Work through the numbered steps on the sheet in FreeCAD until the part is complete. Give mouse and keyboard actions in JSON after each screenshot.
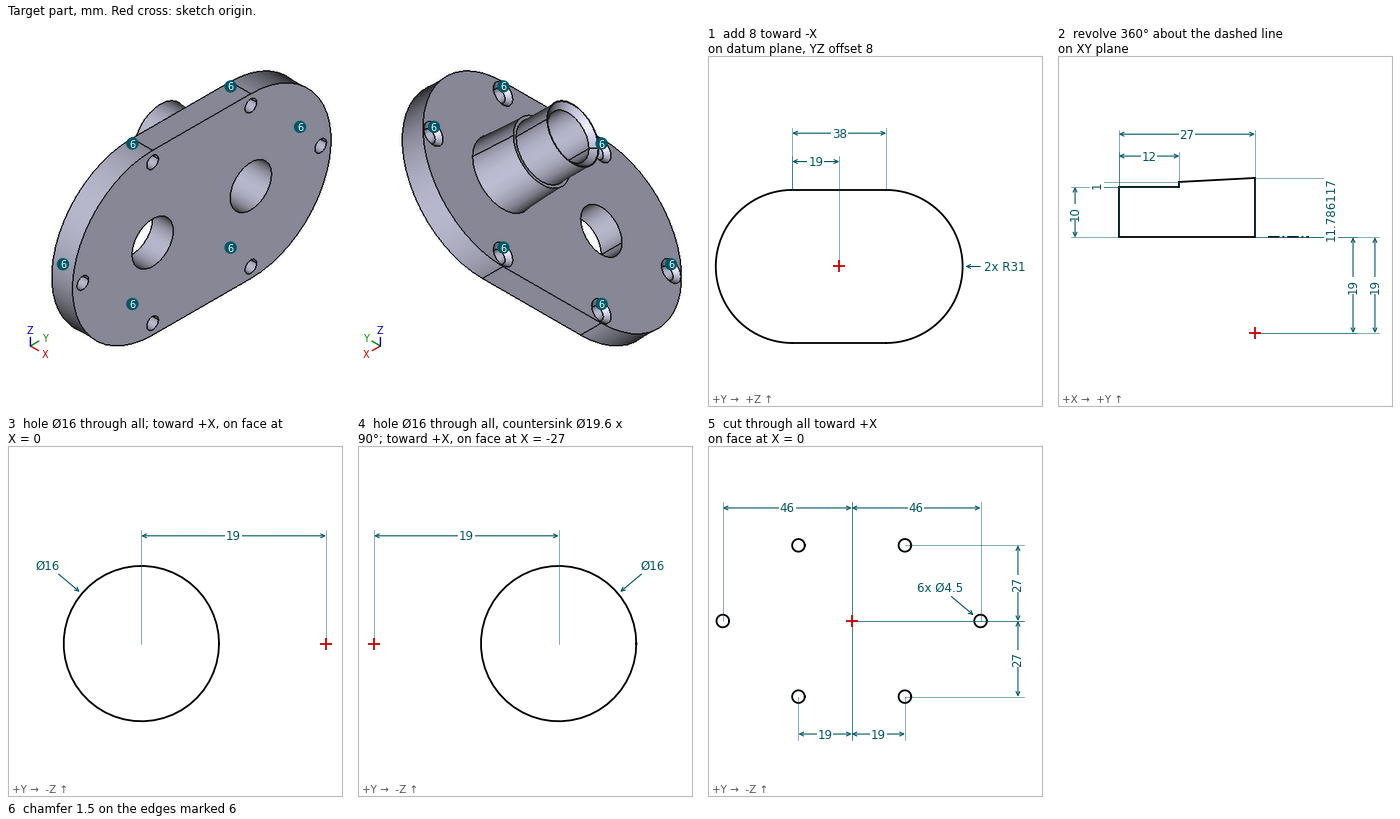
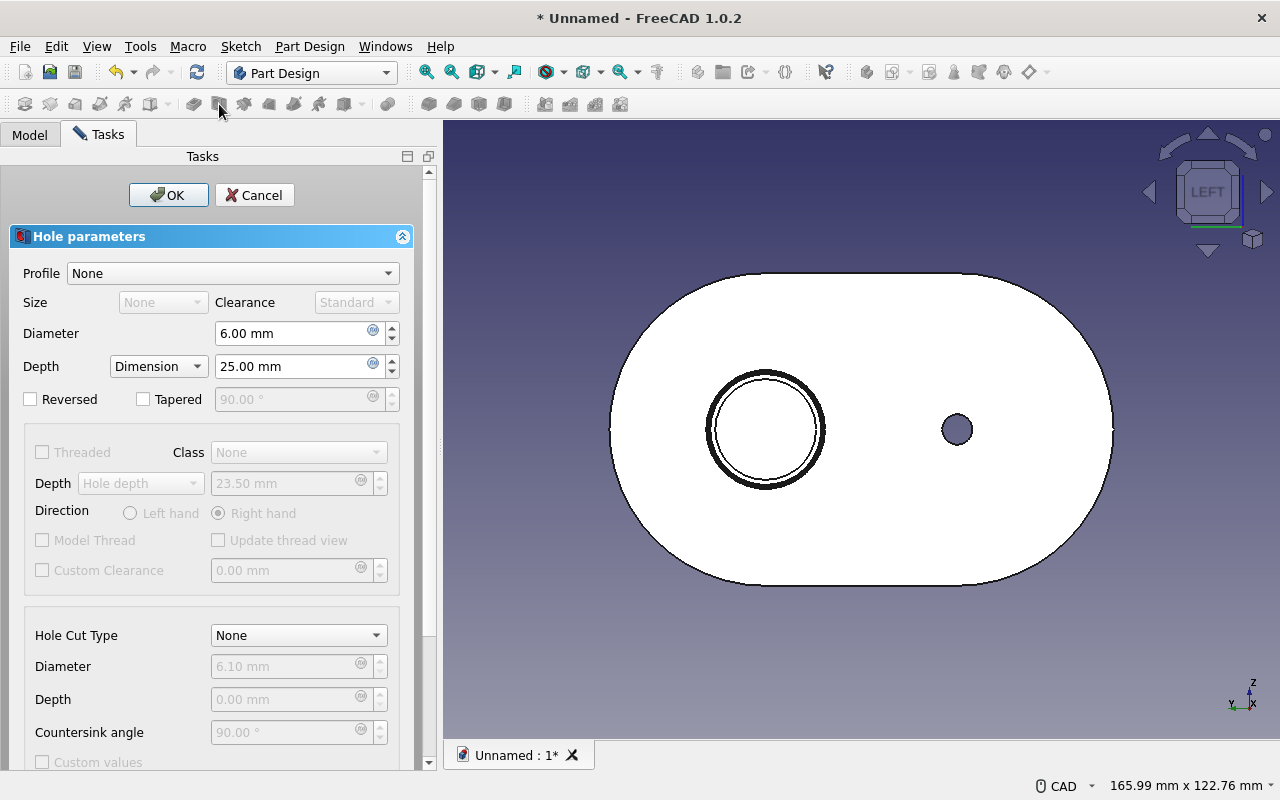
{"action": "triple_click", "coordinate": [300, 334]}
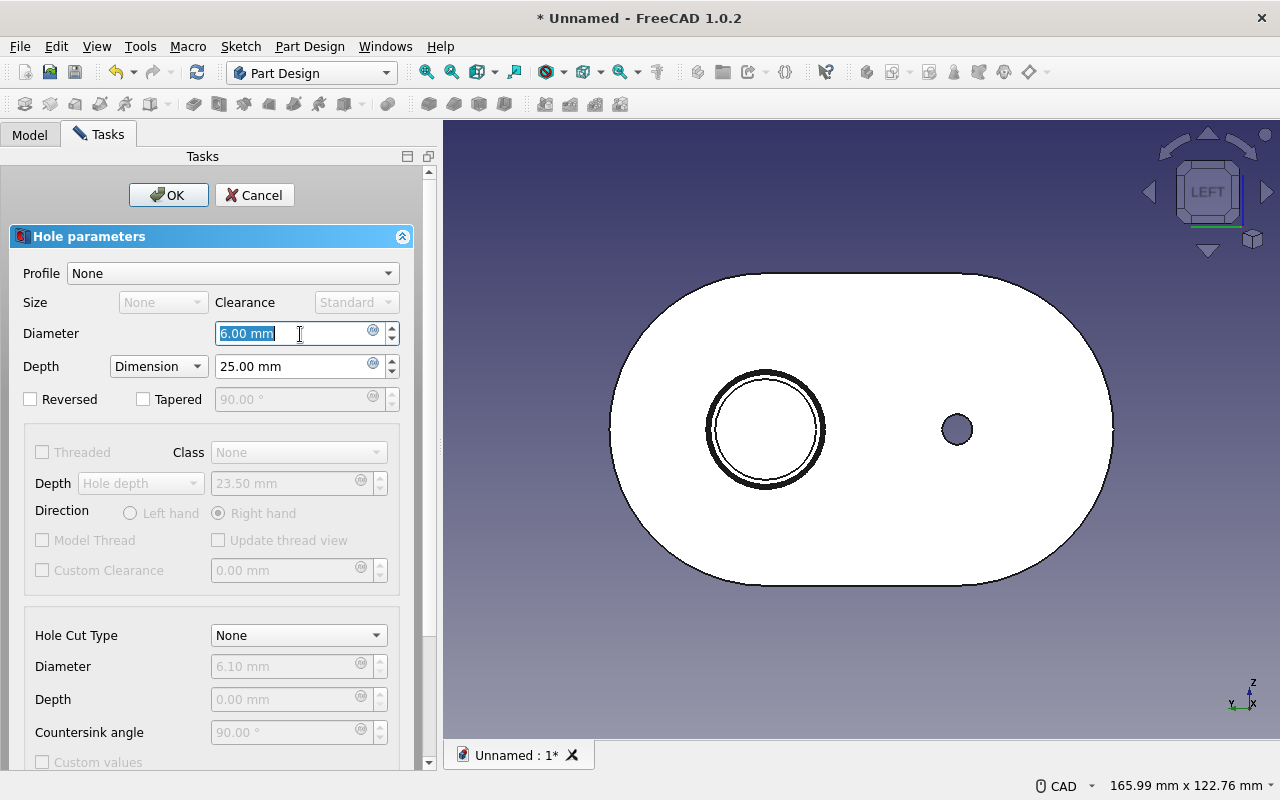
{"action": "type", "text": "16"}
{"action": "key", "text": "Tab"}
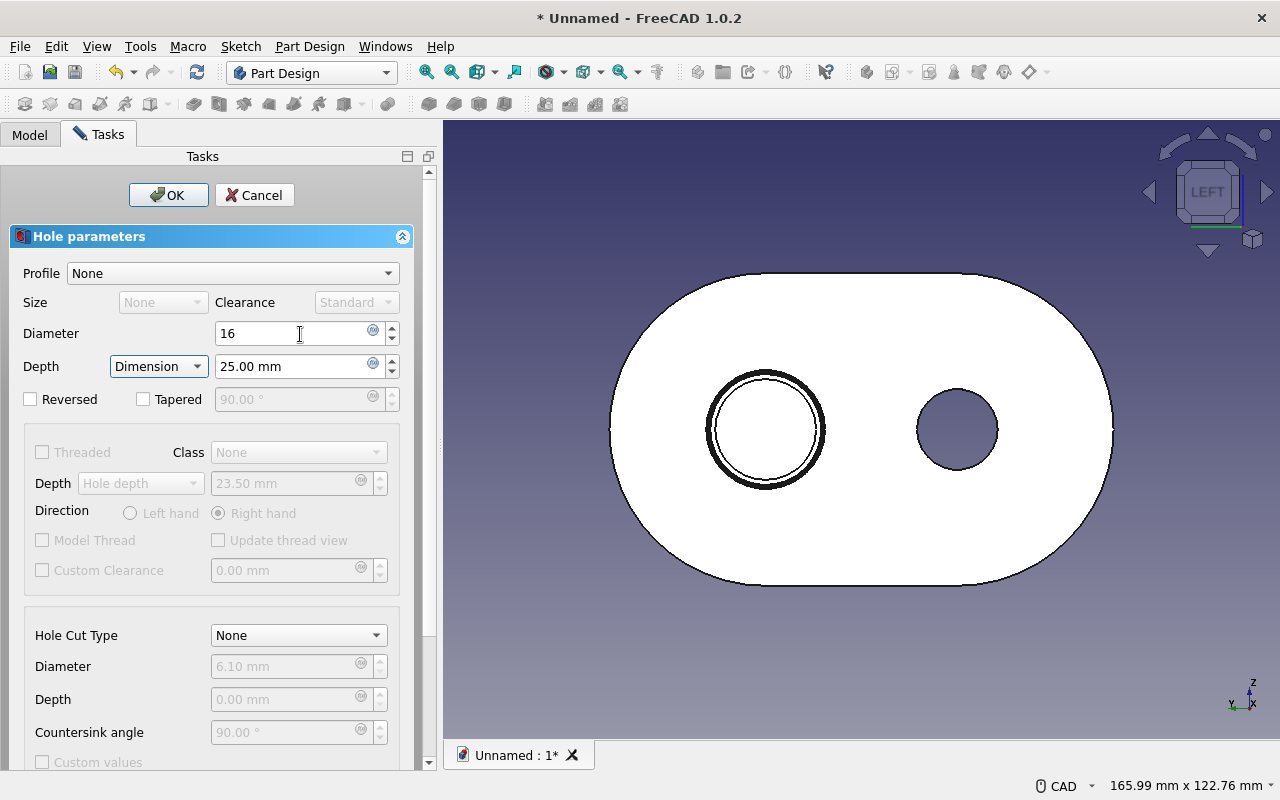
{"action": "left_click", "coordinate": [160, 366]}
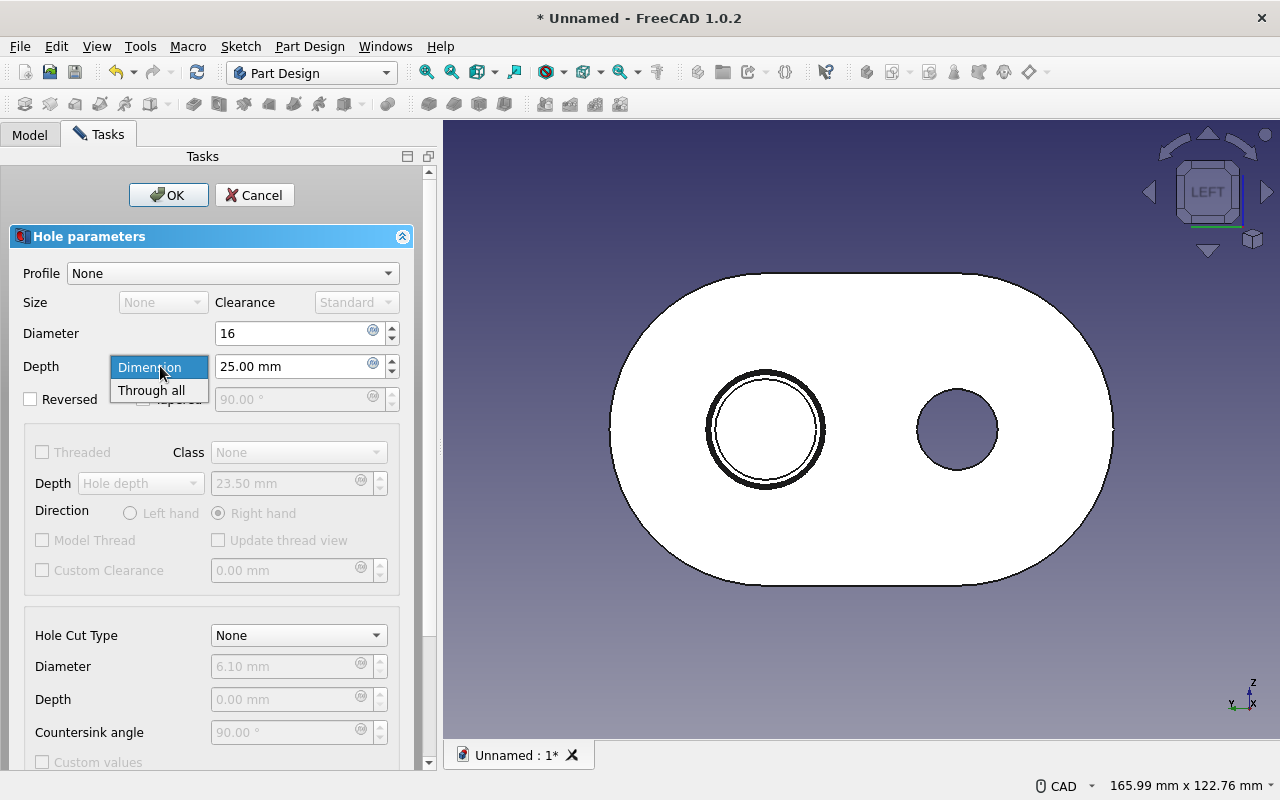
{"action": "left_click", "coordinate": [158, 390]}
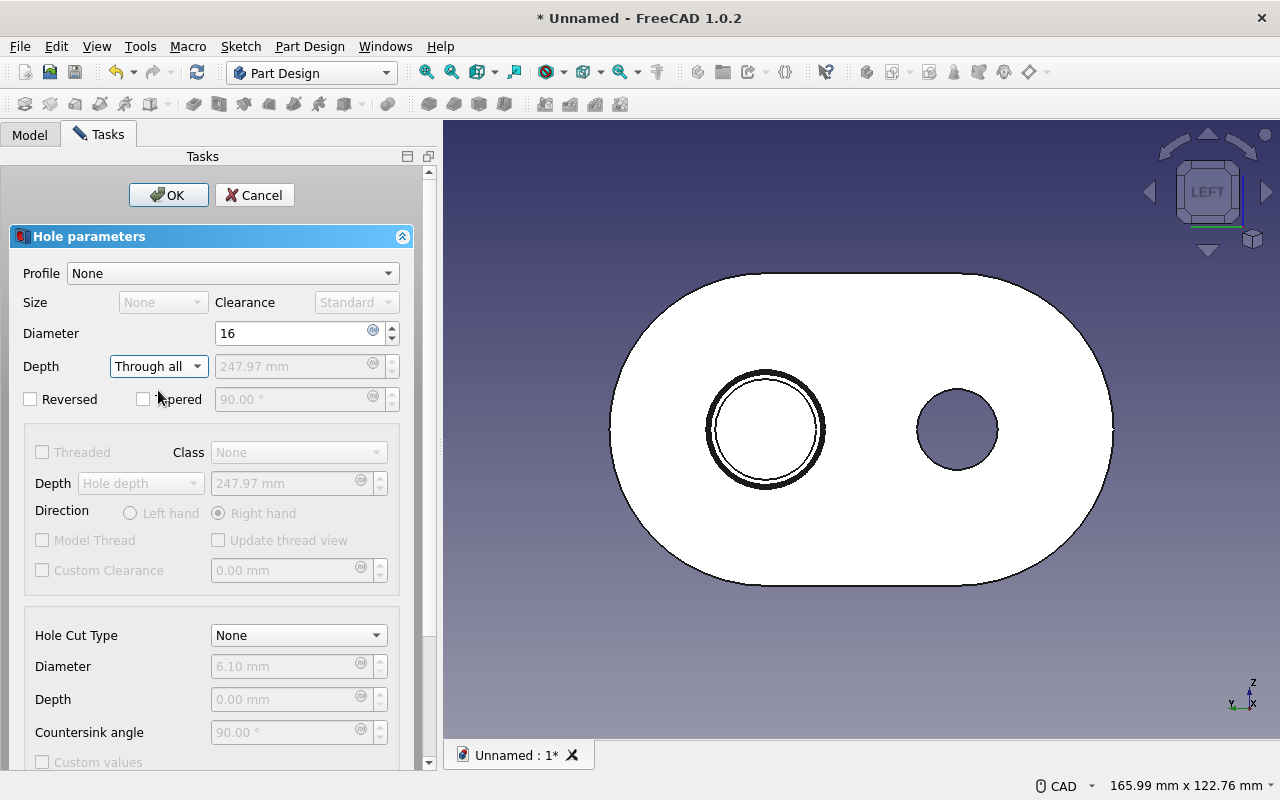
{"action": "left_click", "coordinate": [169, 195]}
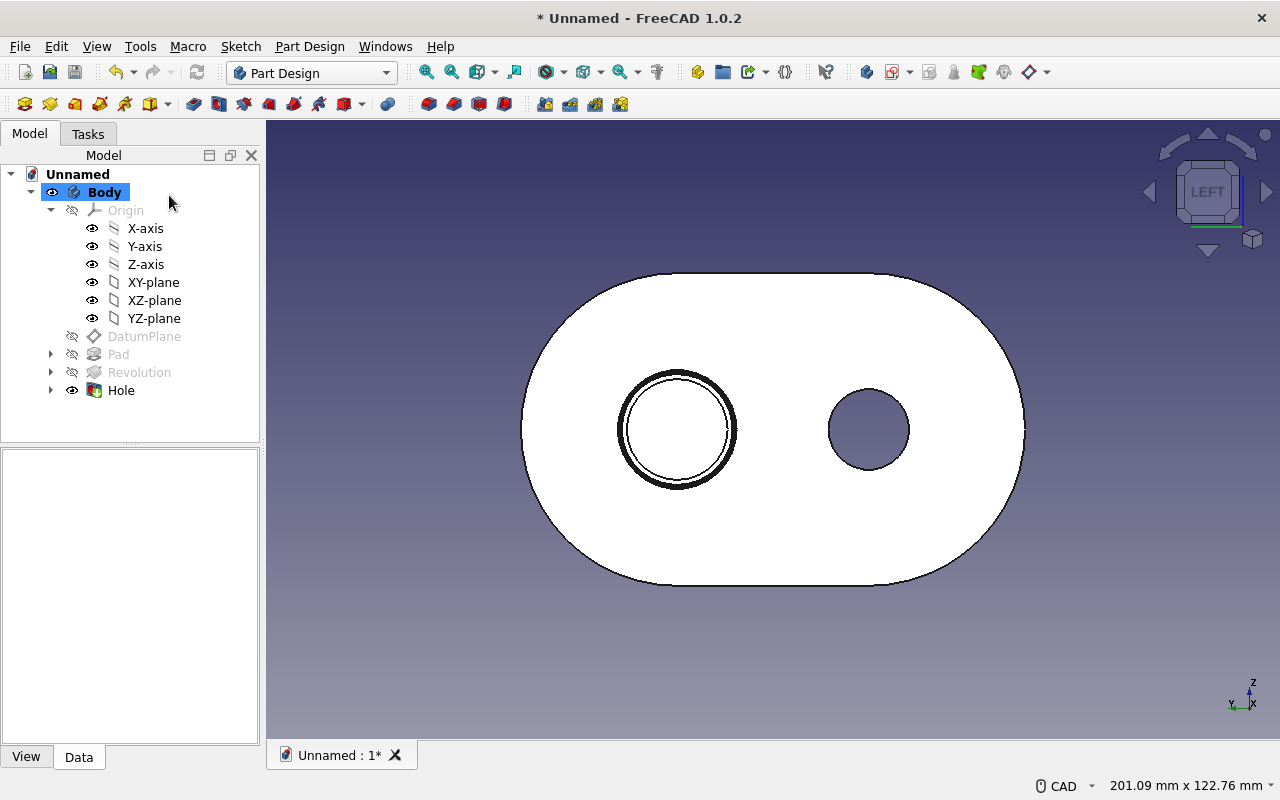
{"action": "left_click", "coordinate": [677, 428]}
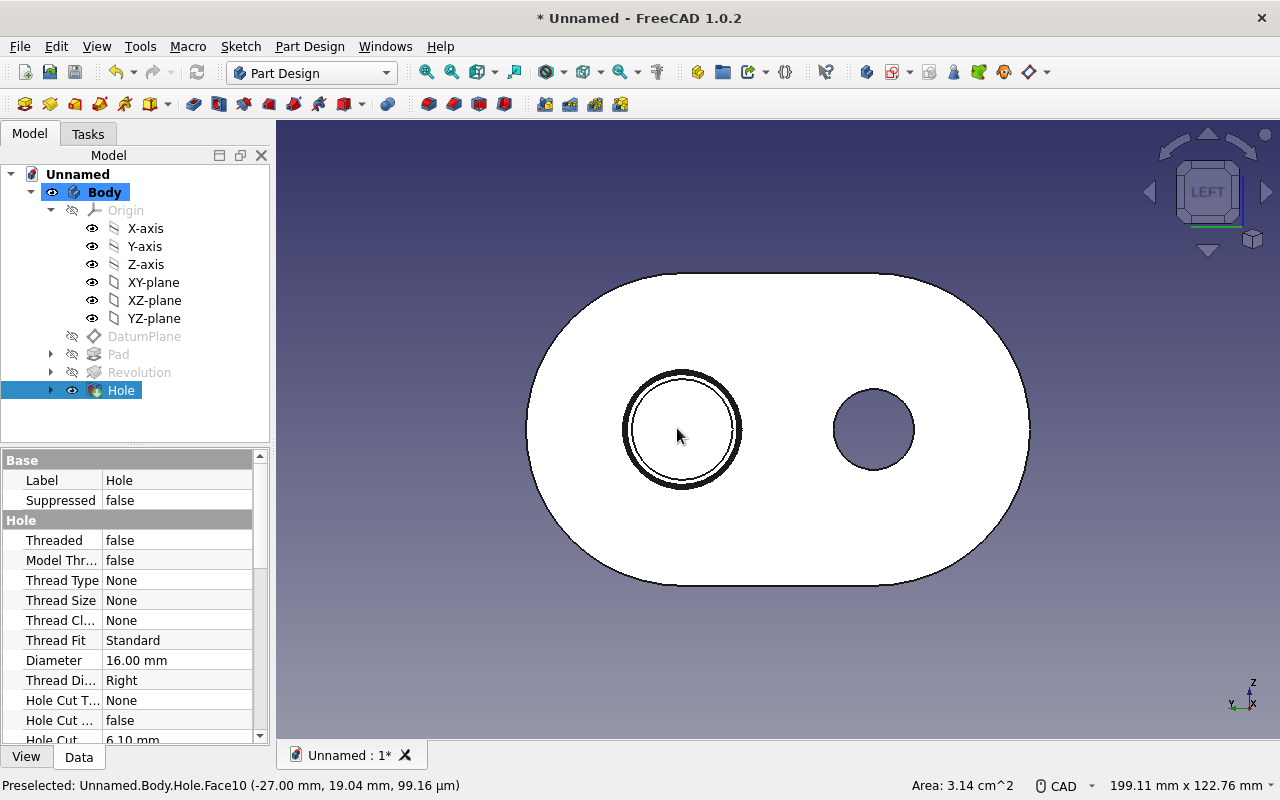
{"action": "left_click", "coordinate": [892, 72]}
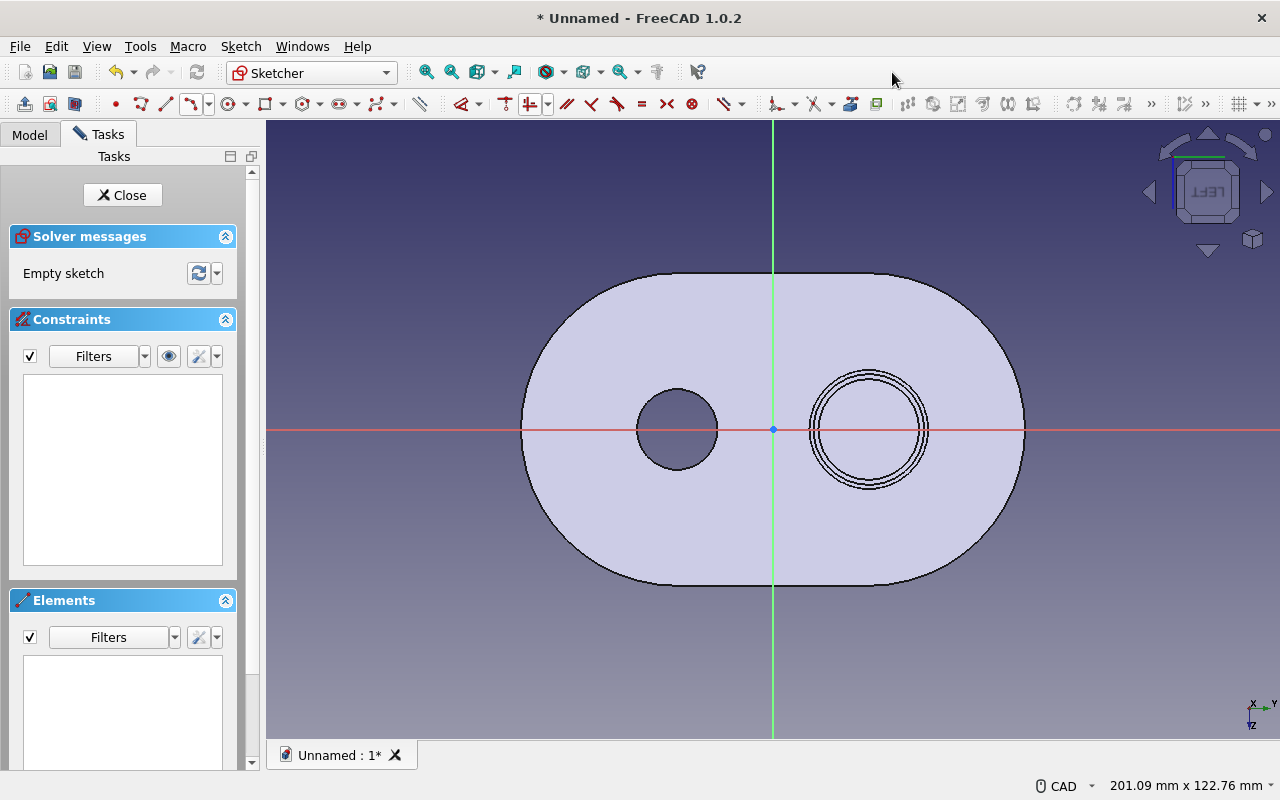
{"action": "scroll", "coordinate": [886, 429], "scroll_direction": "up", "scroll_amount": 7}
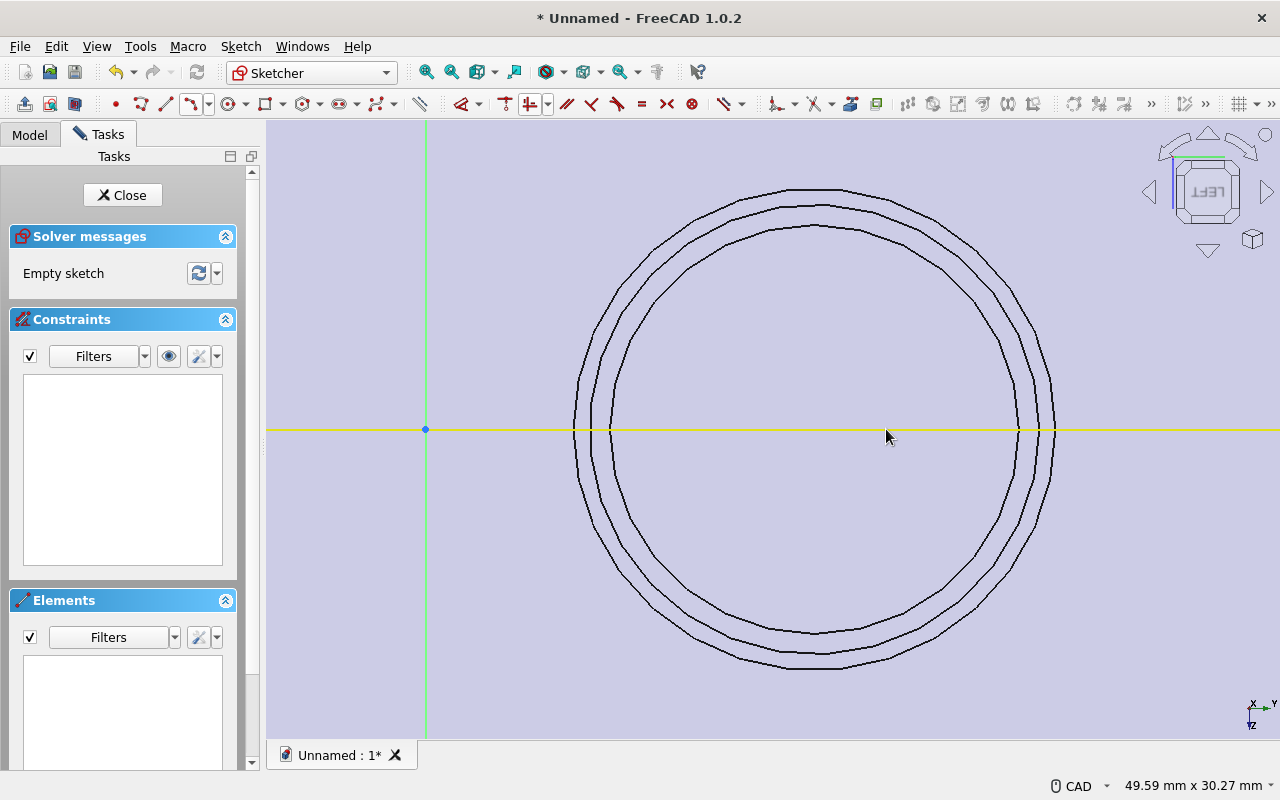
{"action": "key", "text": "g c"}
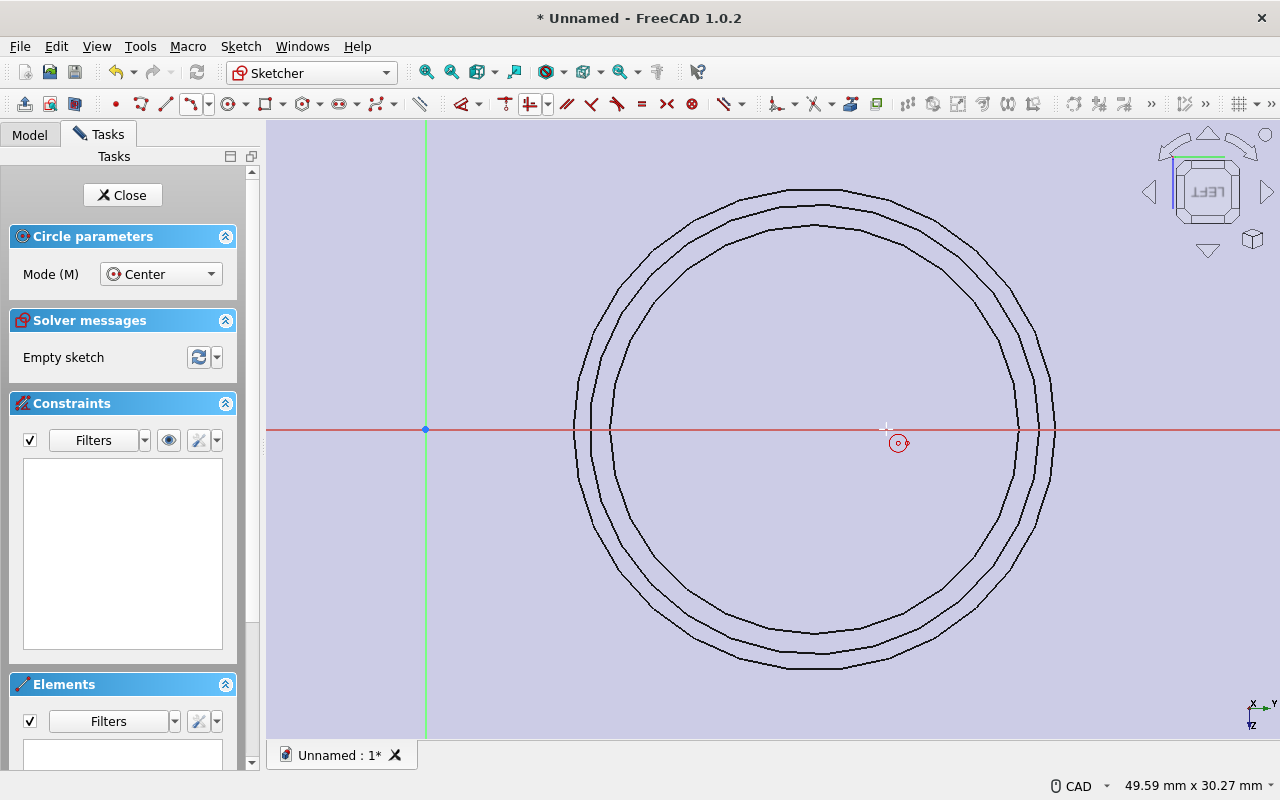
{"action": "left_click", "coordinate": [814, 429]}
{"action": "left_click", "coordinate": [930, 314]}
{"action": "key", "text": "Escape"}